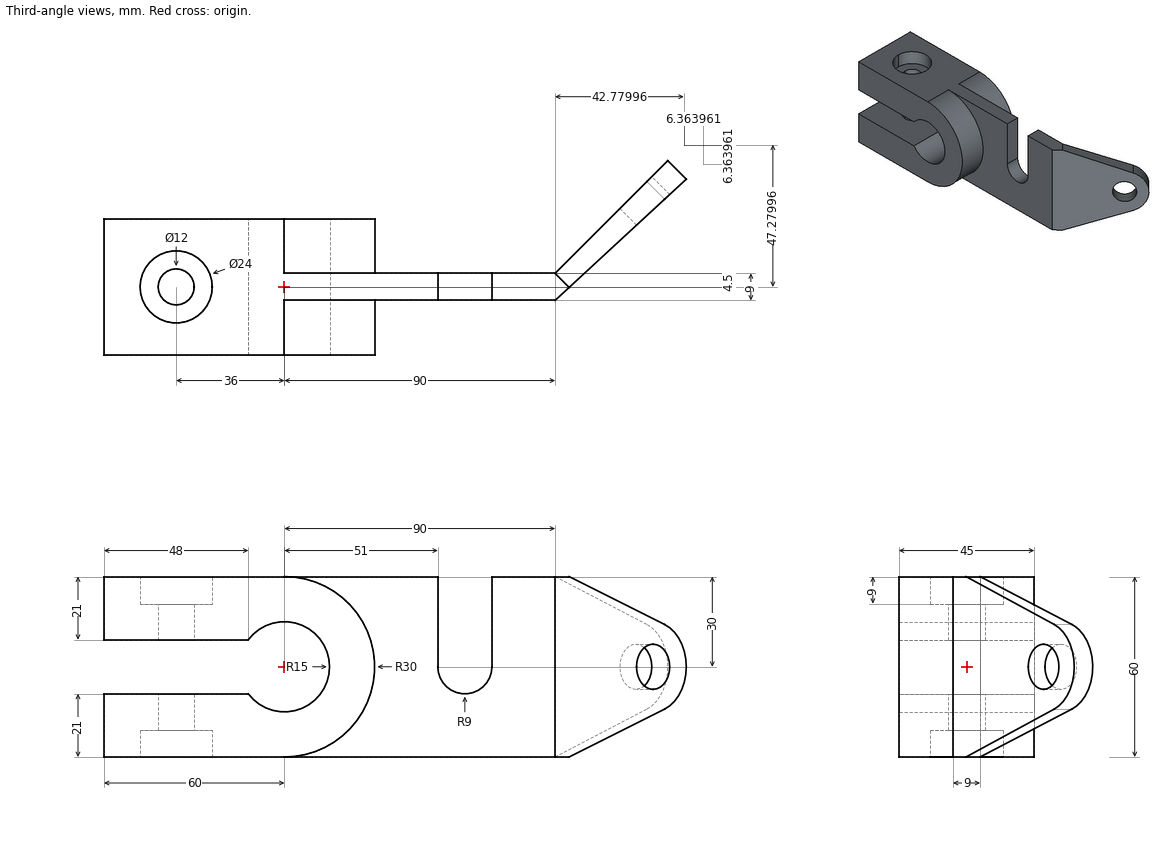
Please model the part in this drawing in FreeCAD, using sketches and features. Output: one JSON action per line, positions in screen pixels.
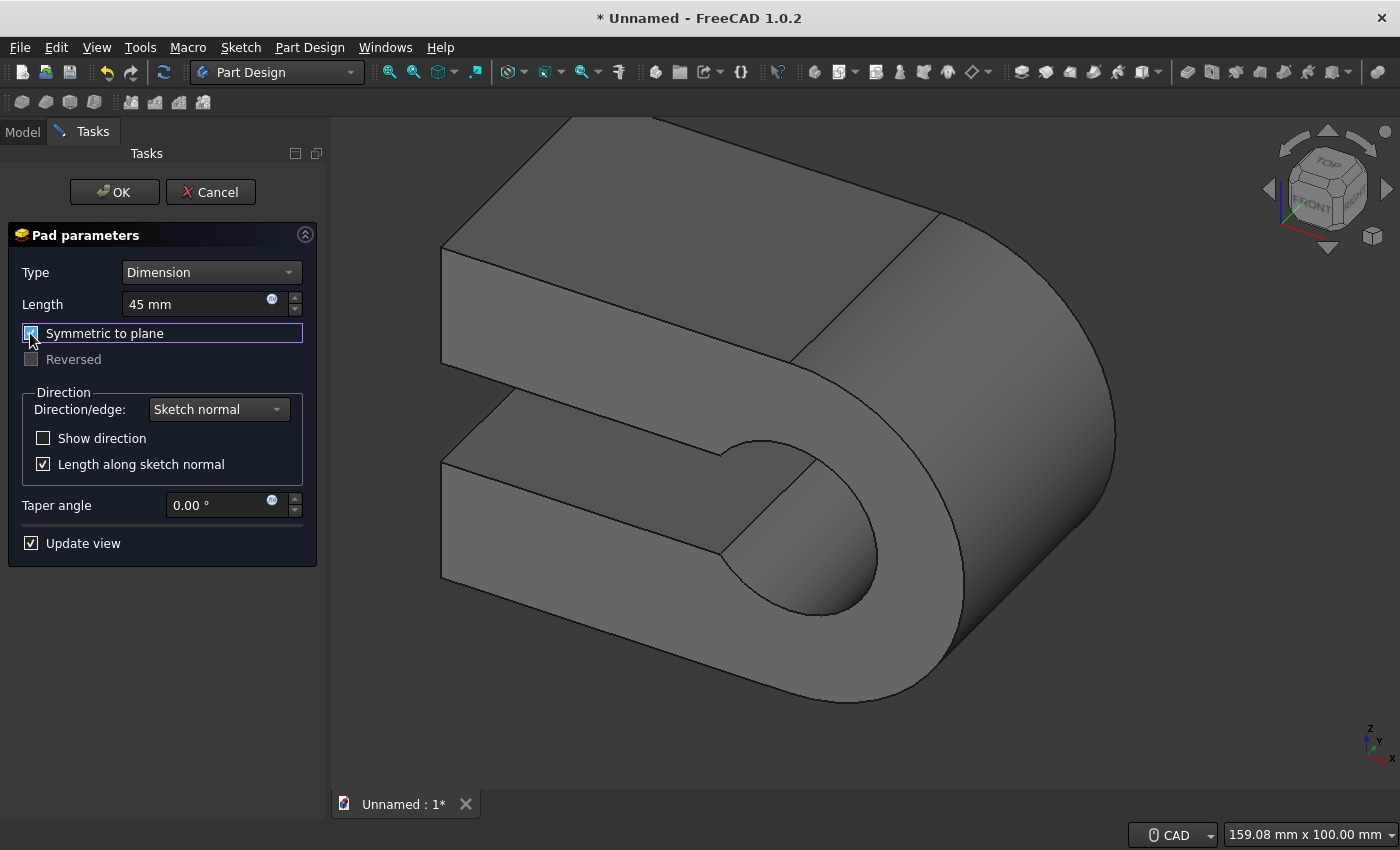
{"action": "left_click", "coordinate": [115, 192]}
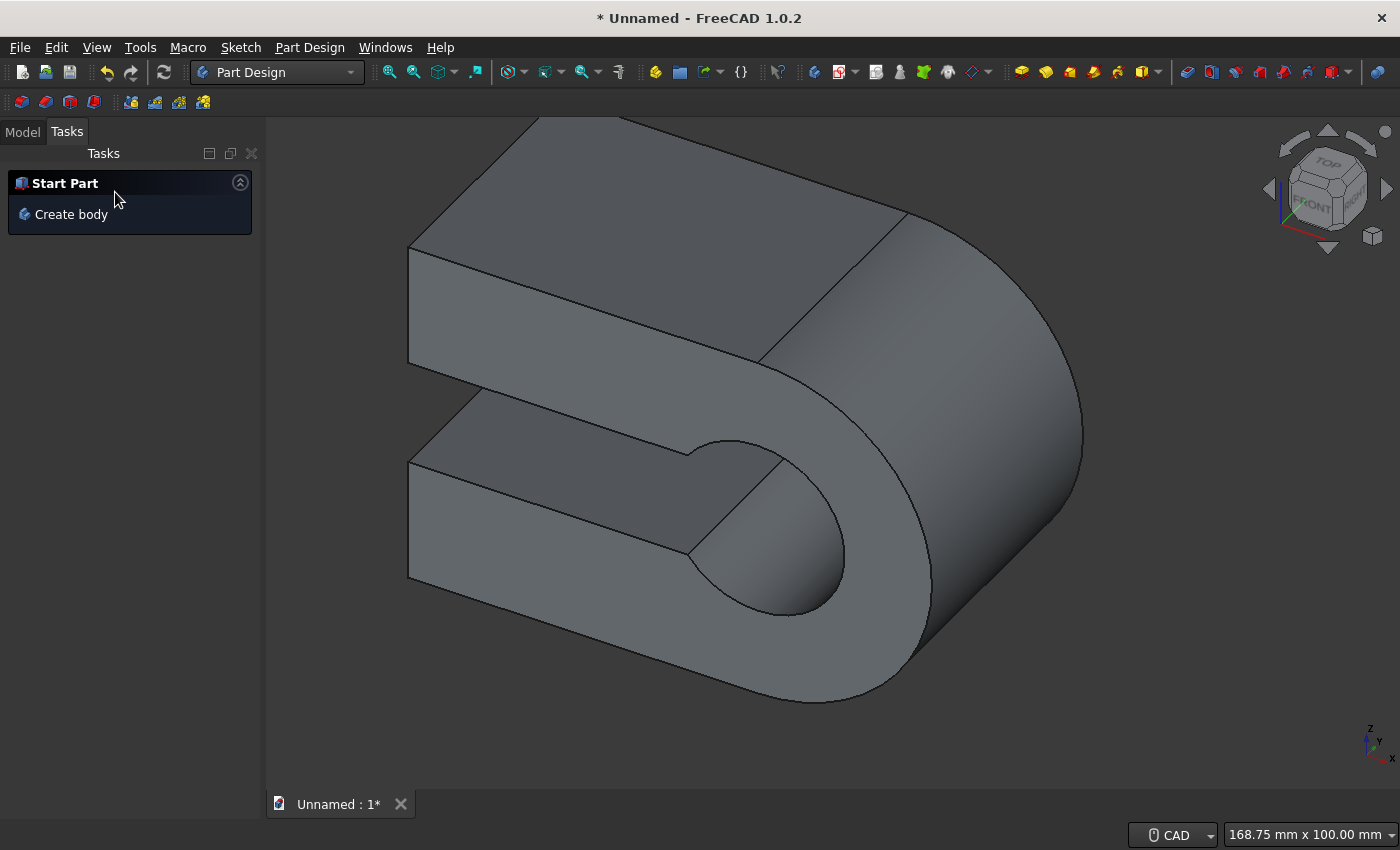
{"action": "key", "text": "v f"}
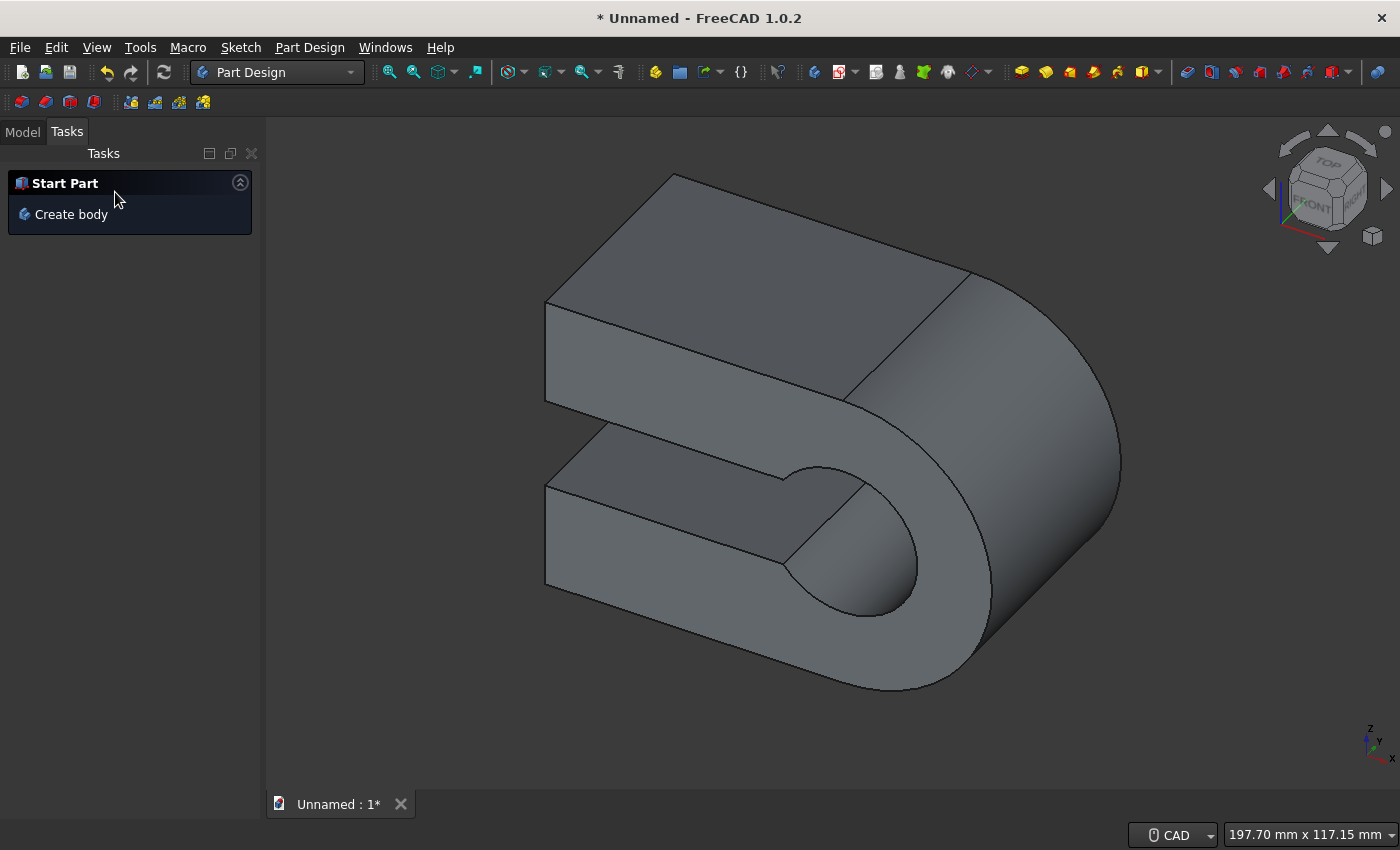
{"action": "left_click", "coordinate": [758, 286]}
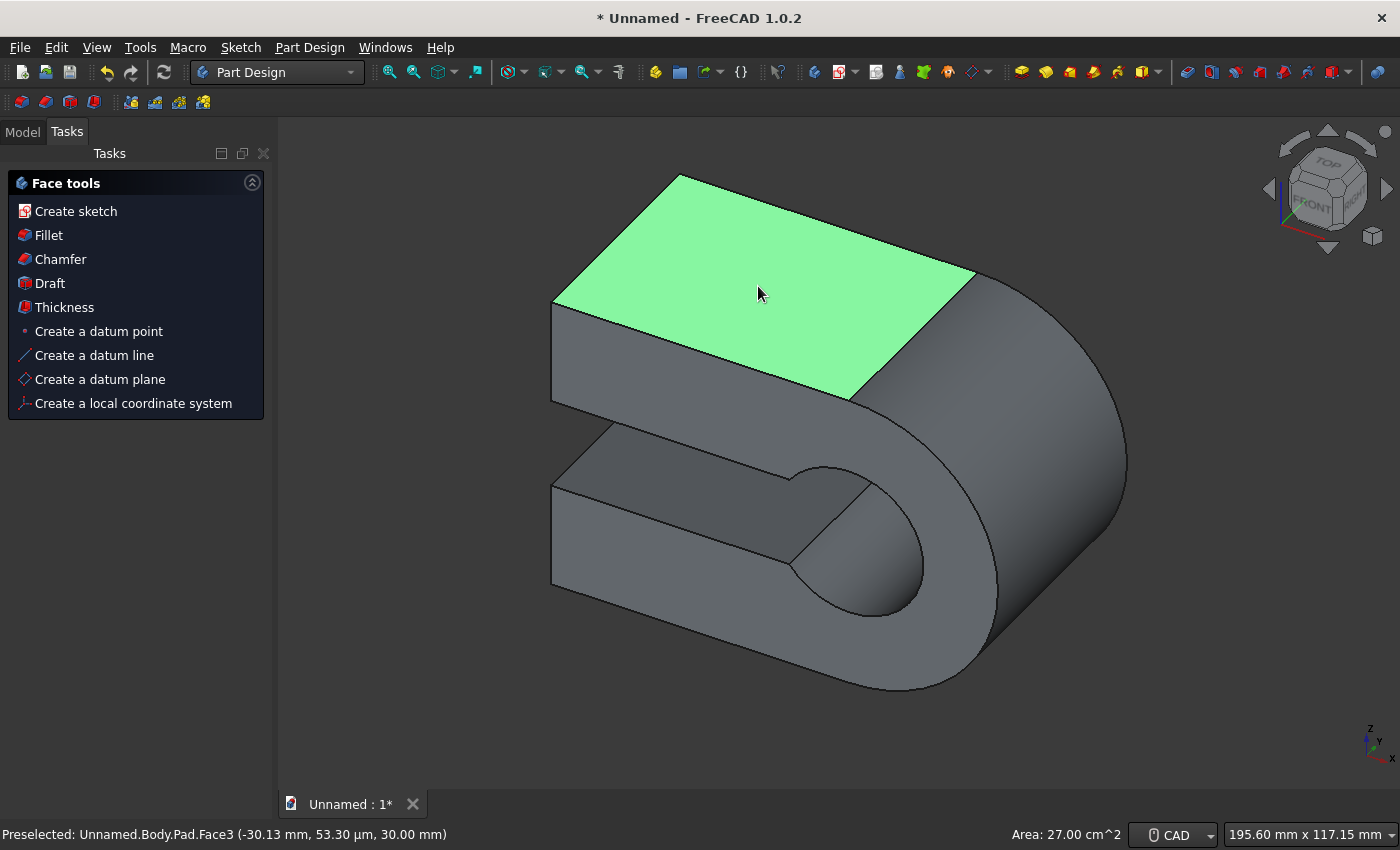
{"action": "left_click", "coordinate": [840, 72]}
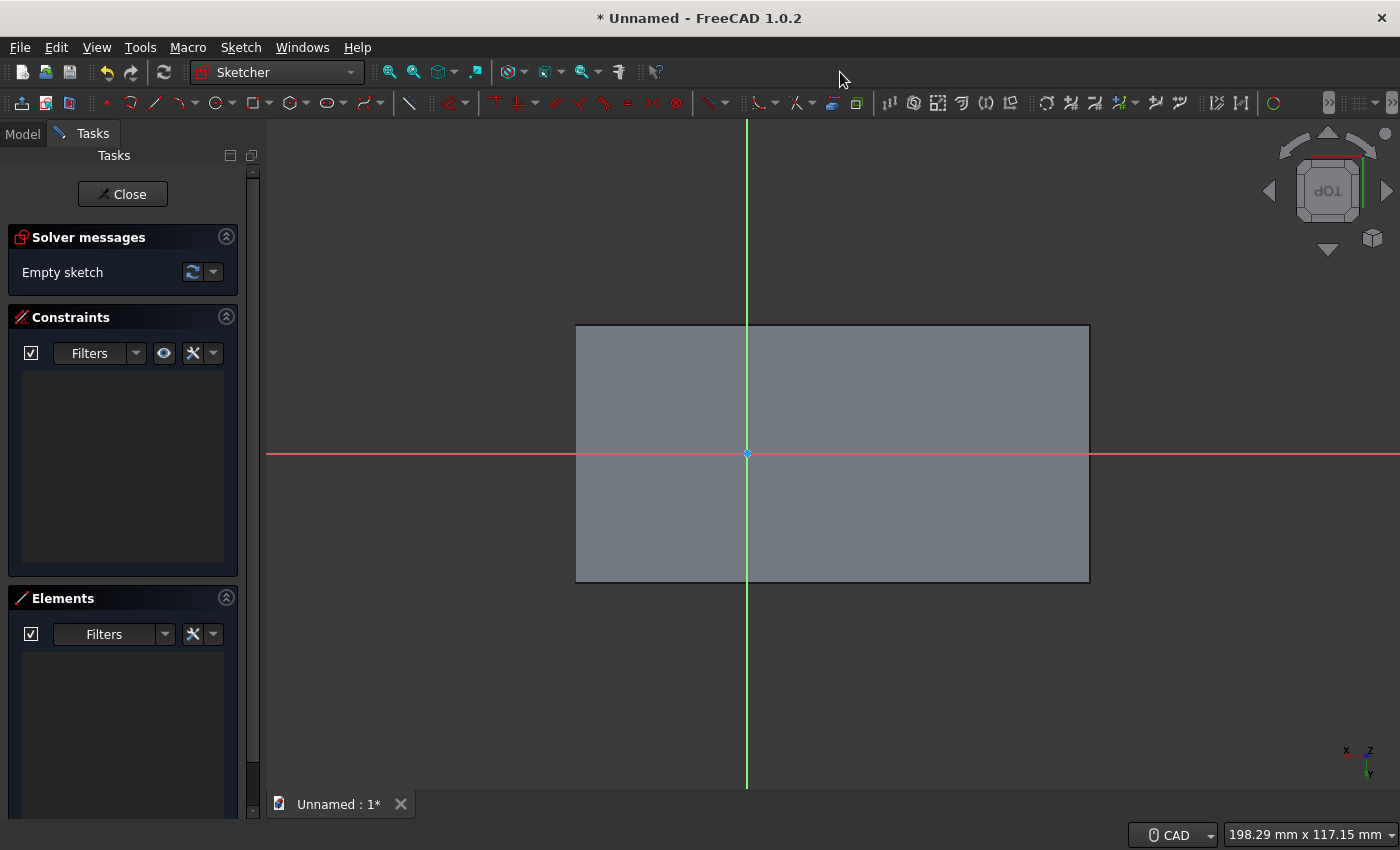
{"action": "scroll", "coordinate": [990, 454], "scroll_direction": "up", "scroll_amount": 9}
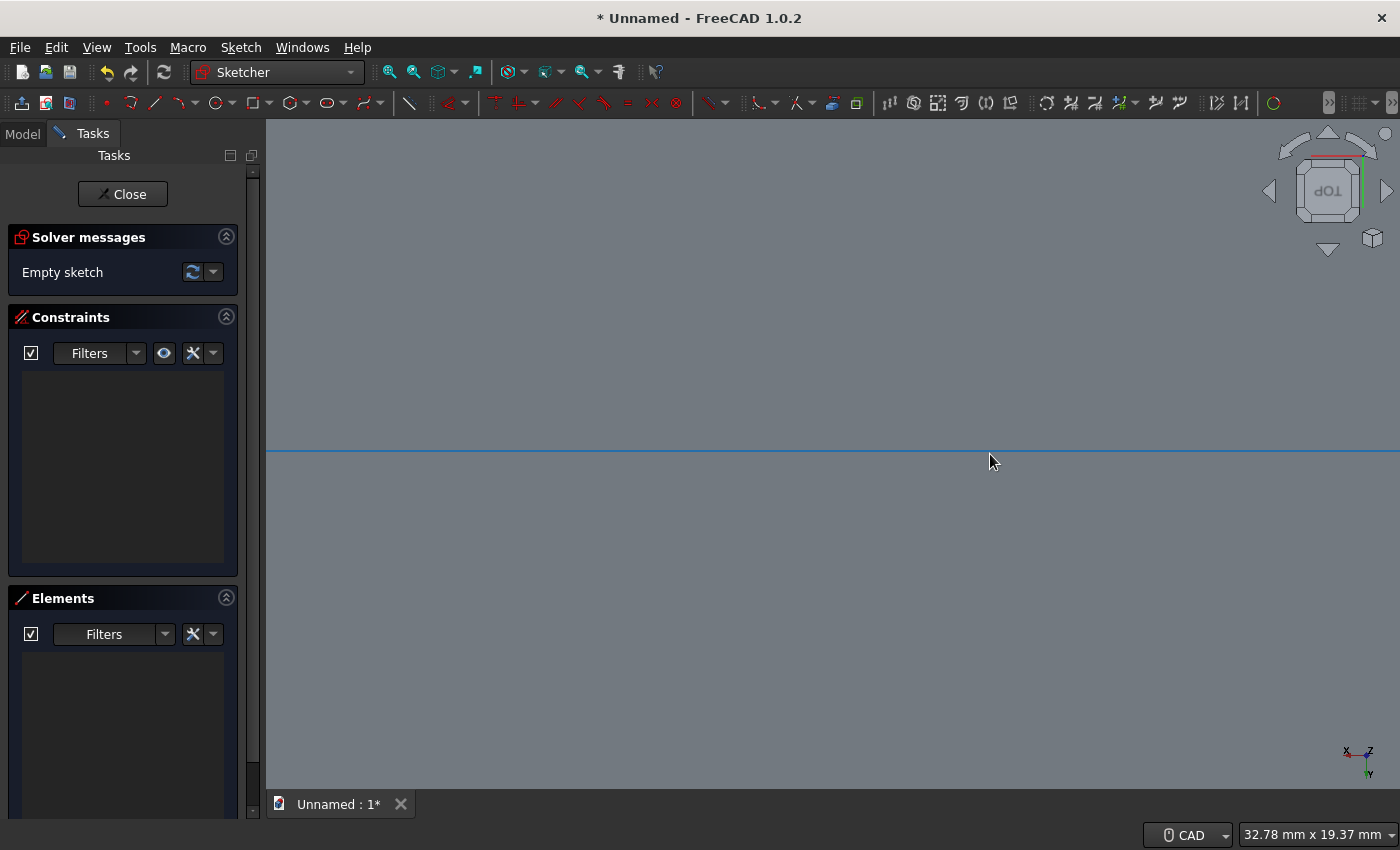
{"action": "key", "text": "g c"}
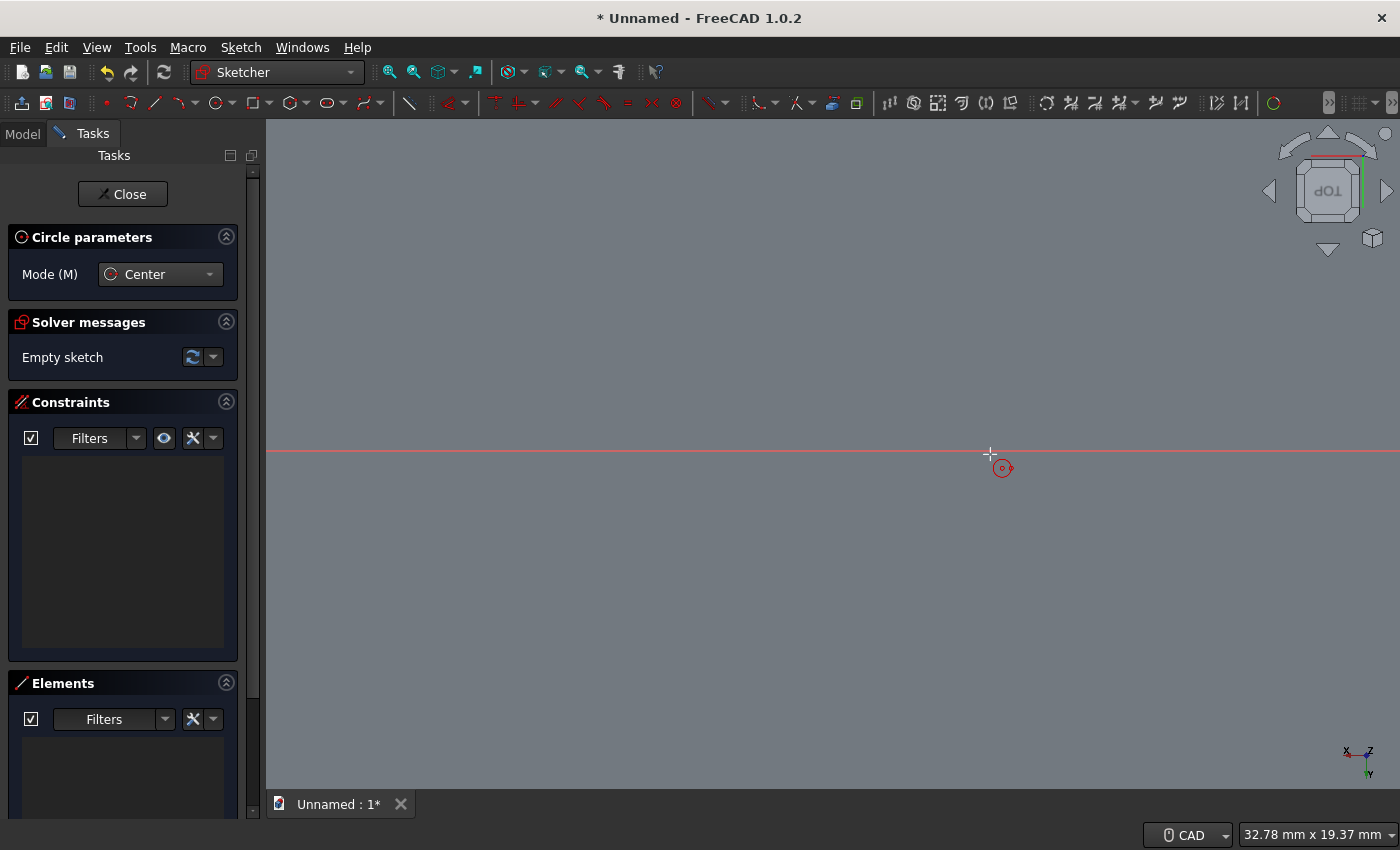
{"action": "left_click", "coordinate": [764, 451]}
{"action": "left_click", "coordinate": [910, 305]}
{"action": "key", "text": "Escape"}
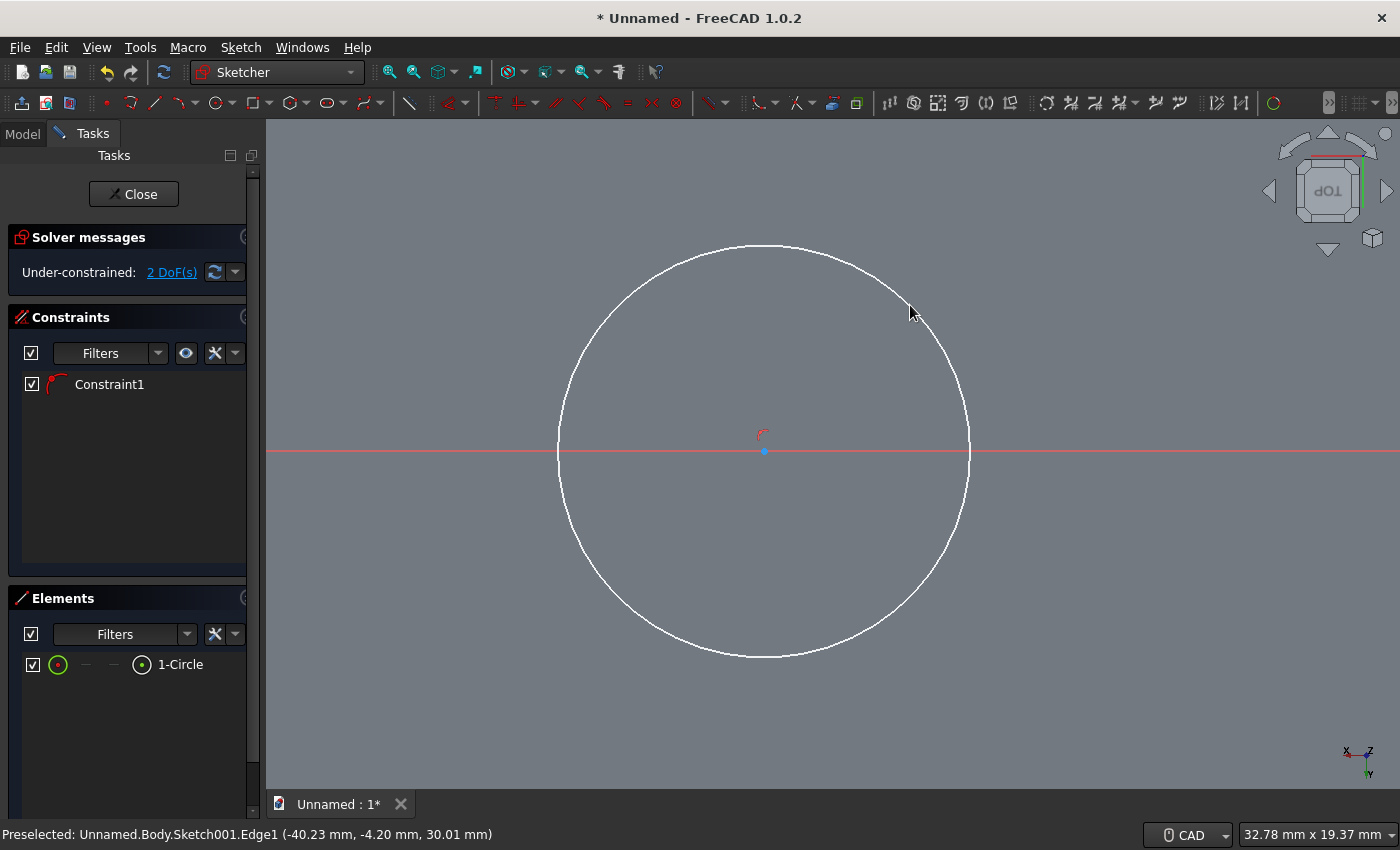
{"action": "key", "text": "d"}